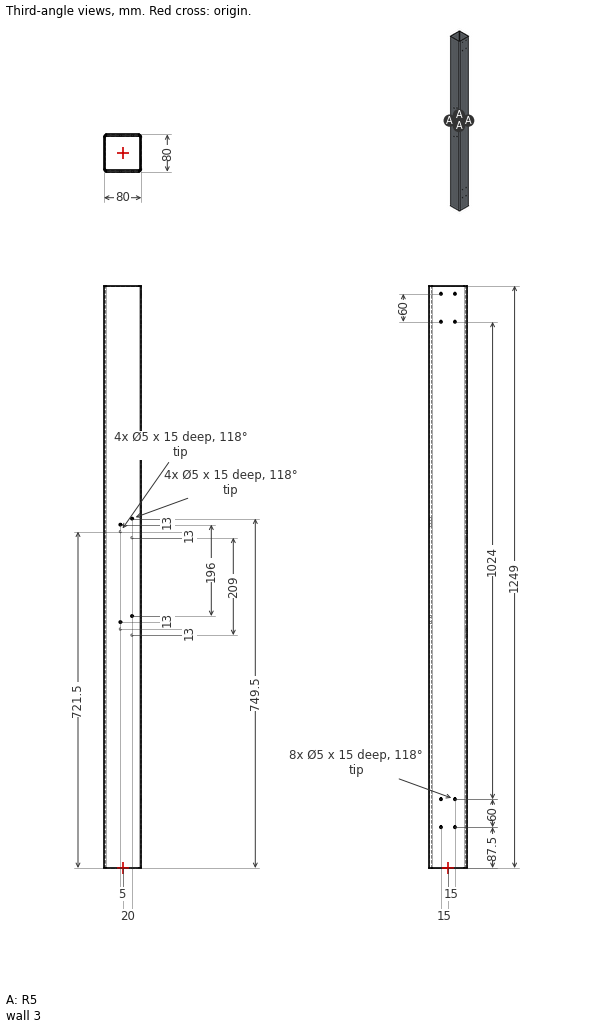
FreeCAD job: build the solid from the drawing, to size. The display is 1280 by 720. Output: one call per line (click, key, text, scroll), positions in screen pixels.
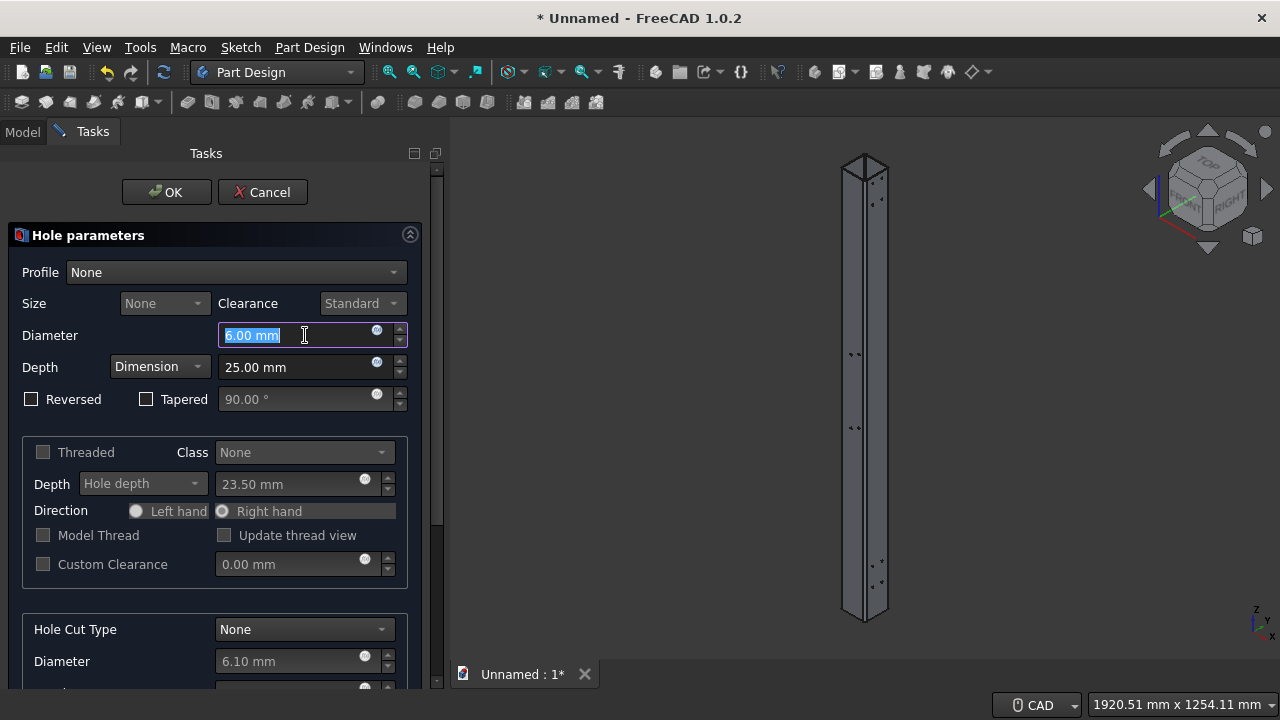
text(5)
key(Tab)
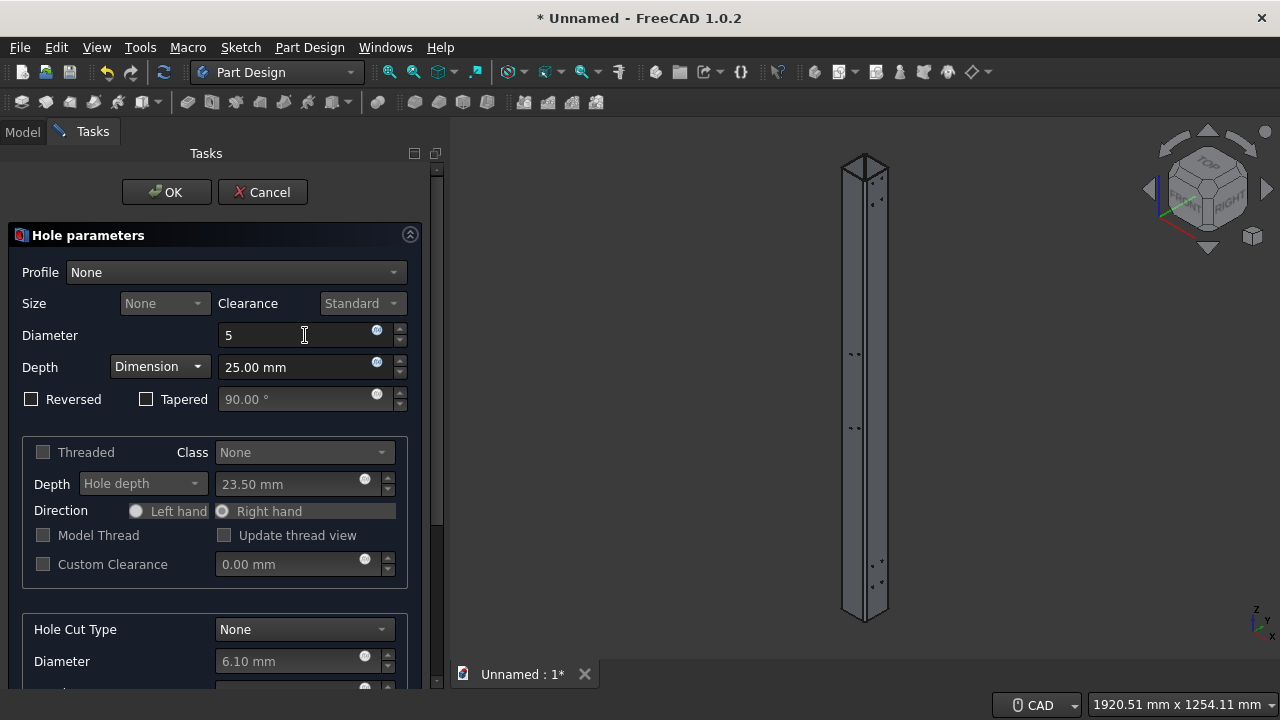
triple_click(305, 367)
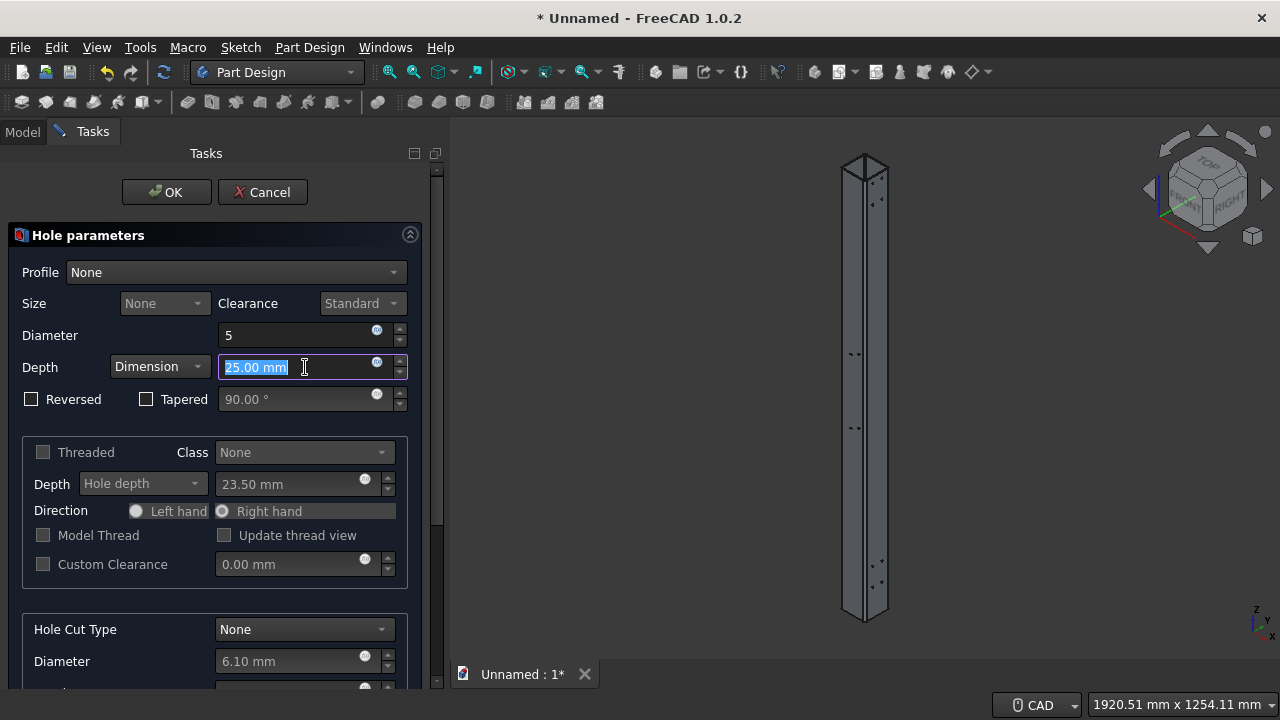
text(15)
key(Tab)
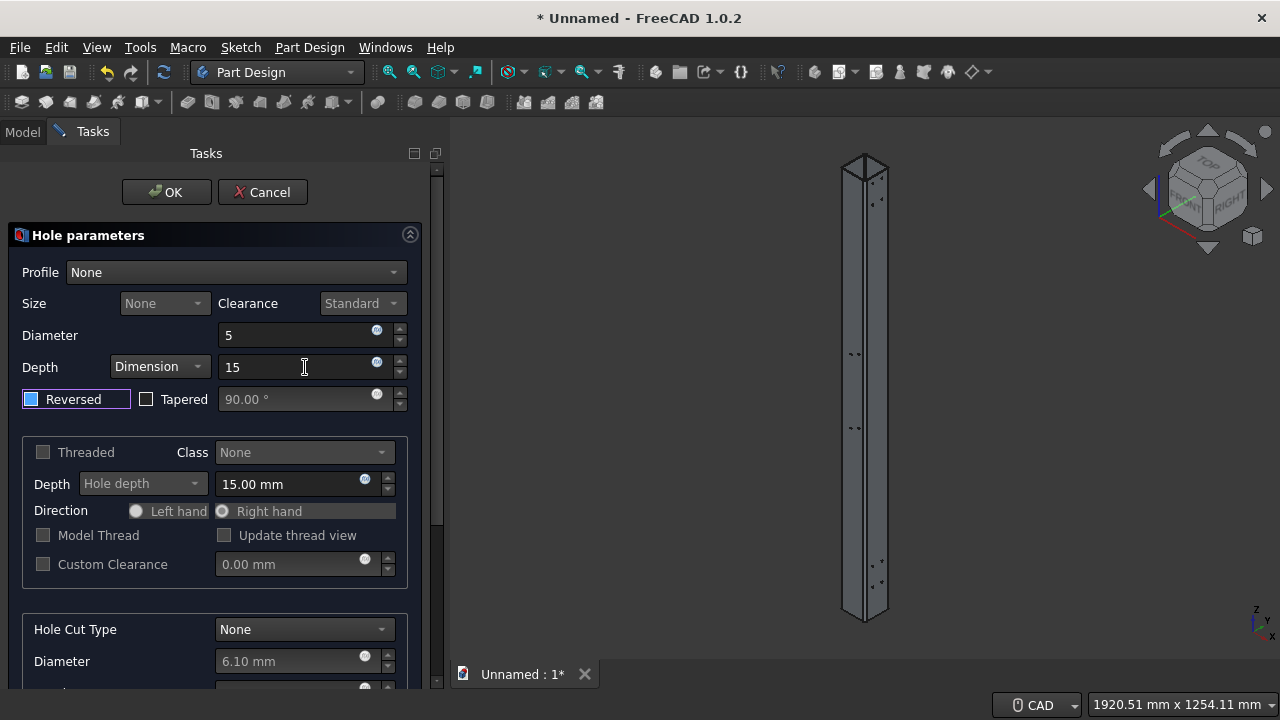
click(167, 192)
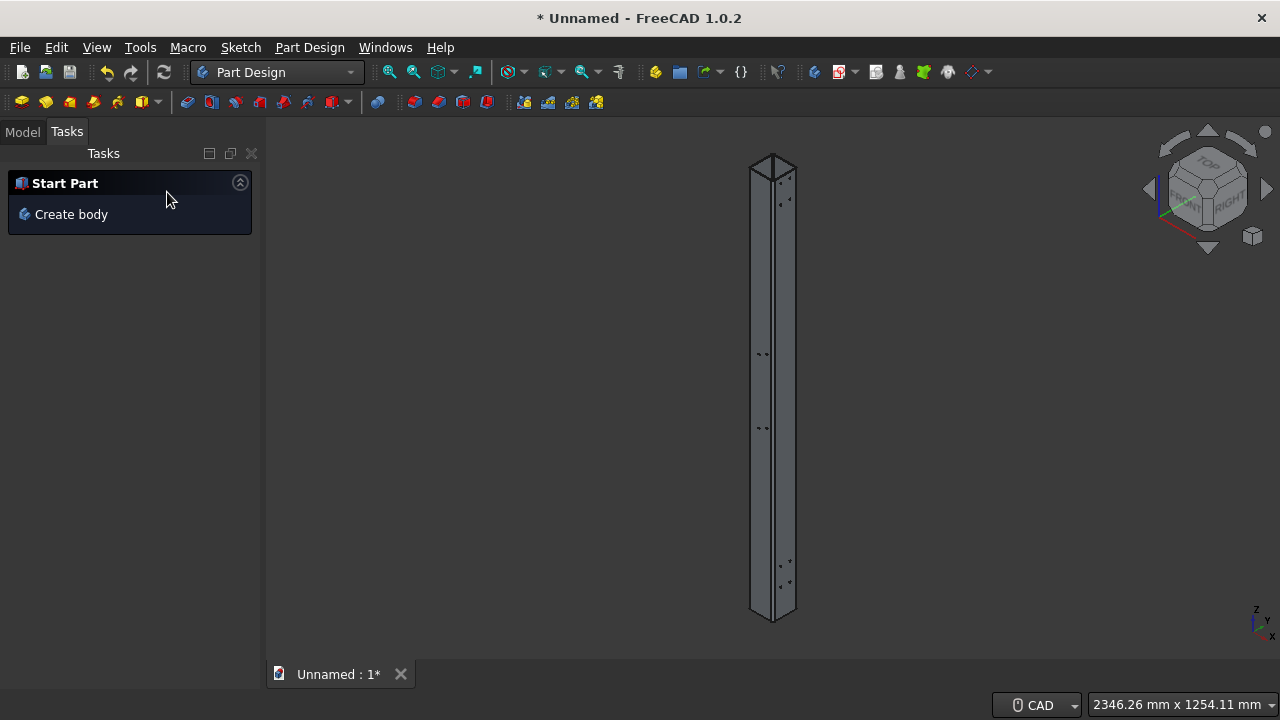
key(4)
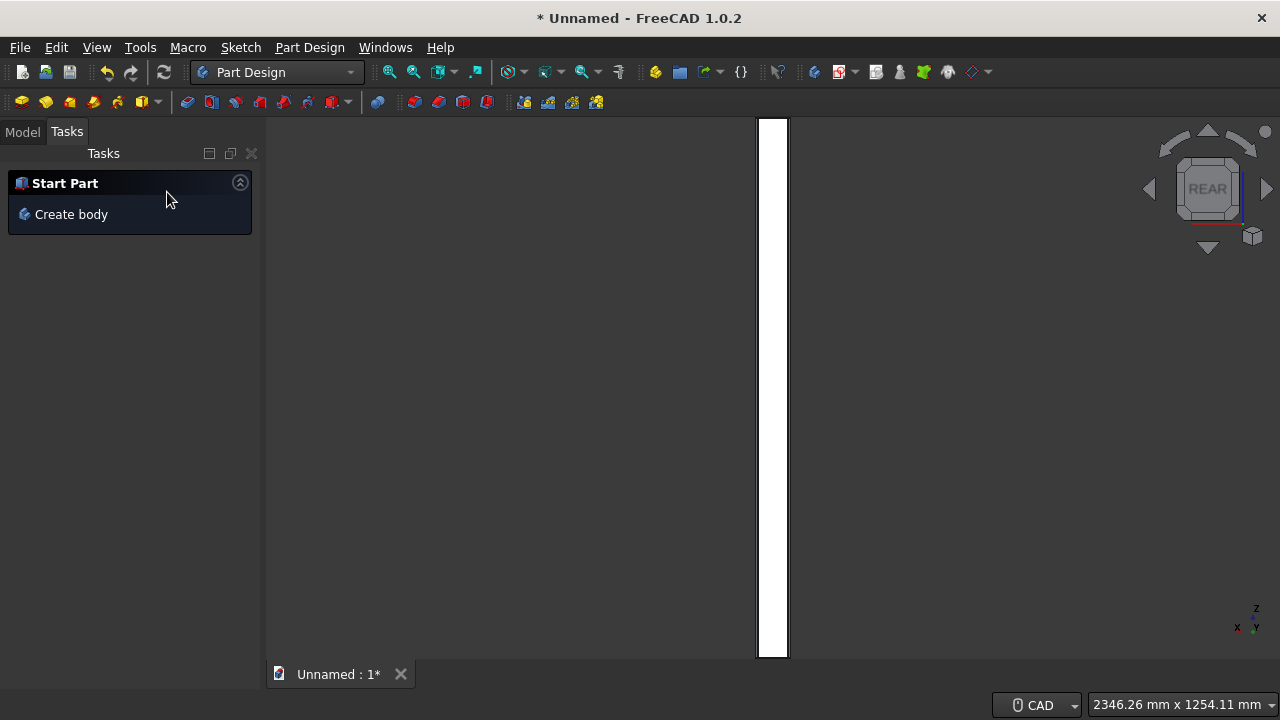
click(773, 156)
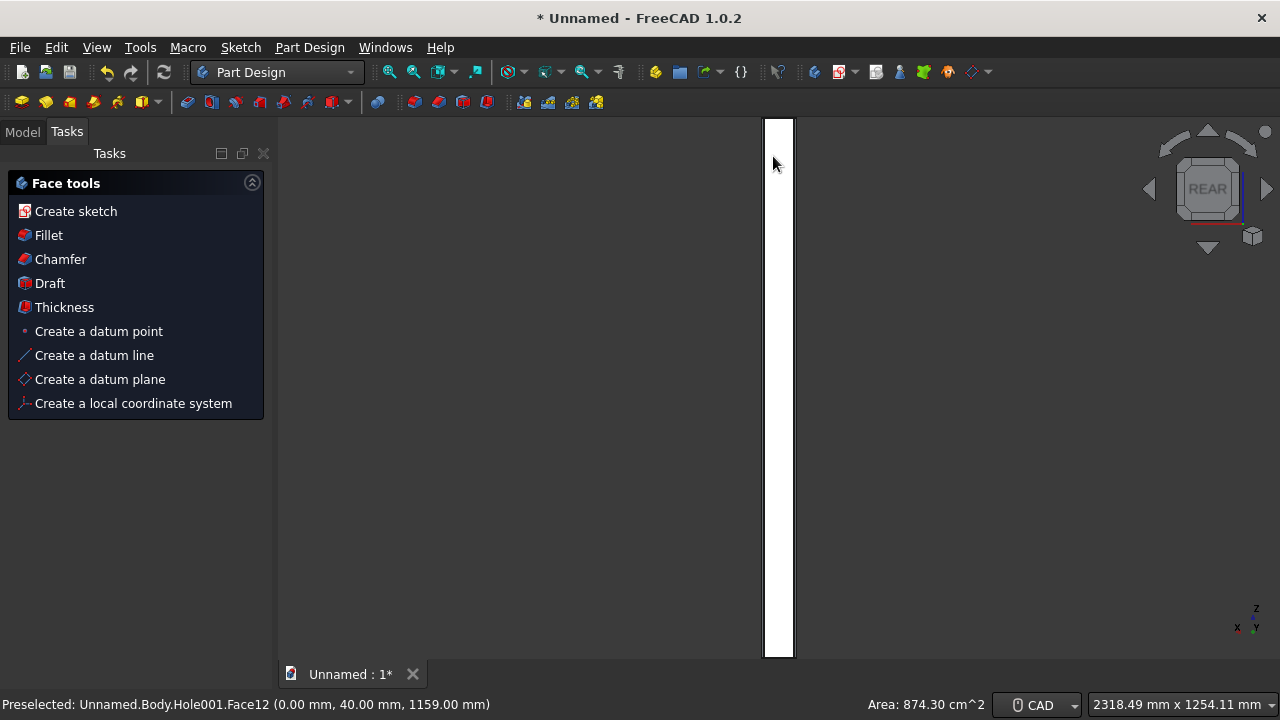
click(840, 72)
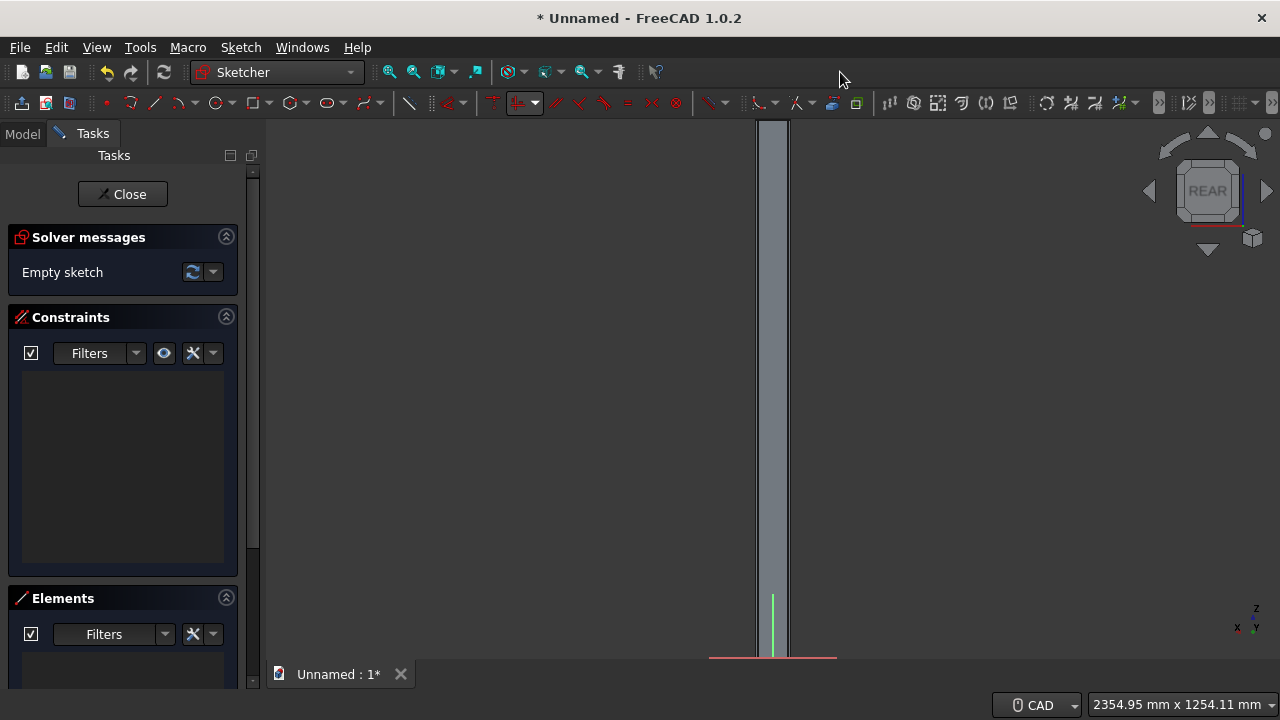
scroll(798, 398, up, 6)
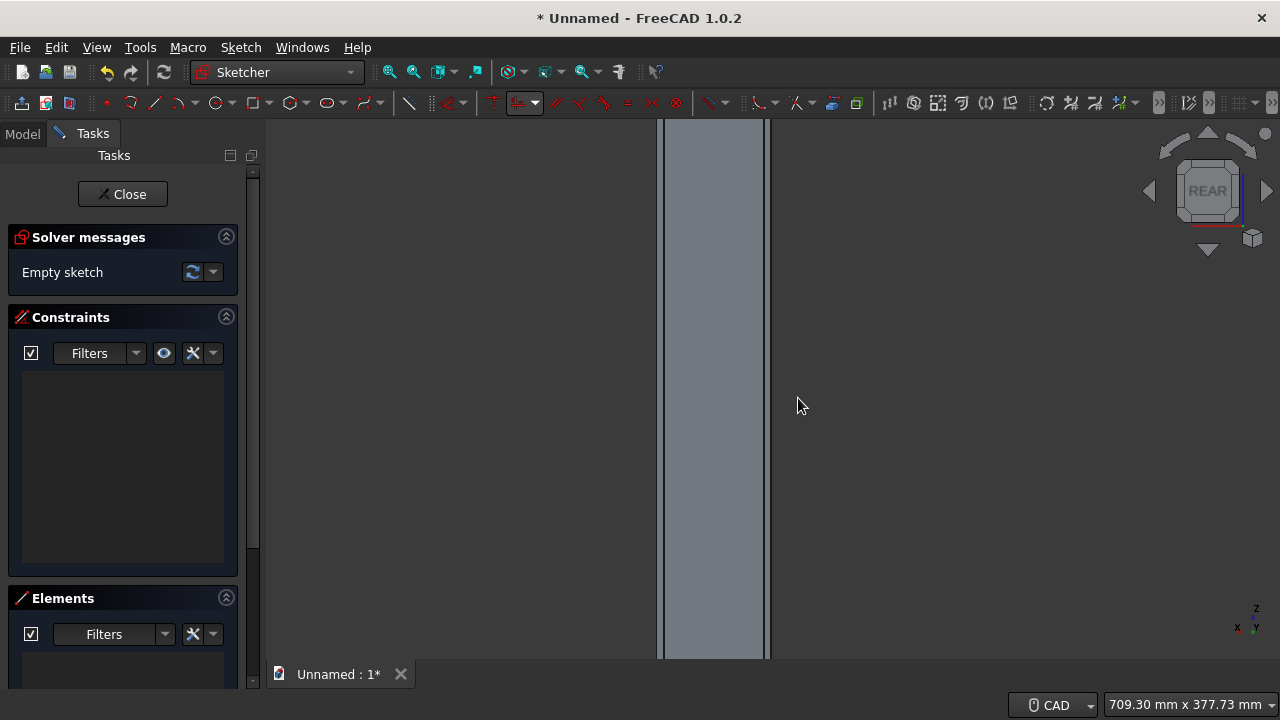
key(g)
key(c)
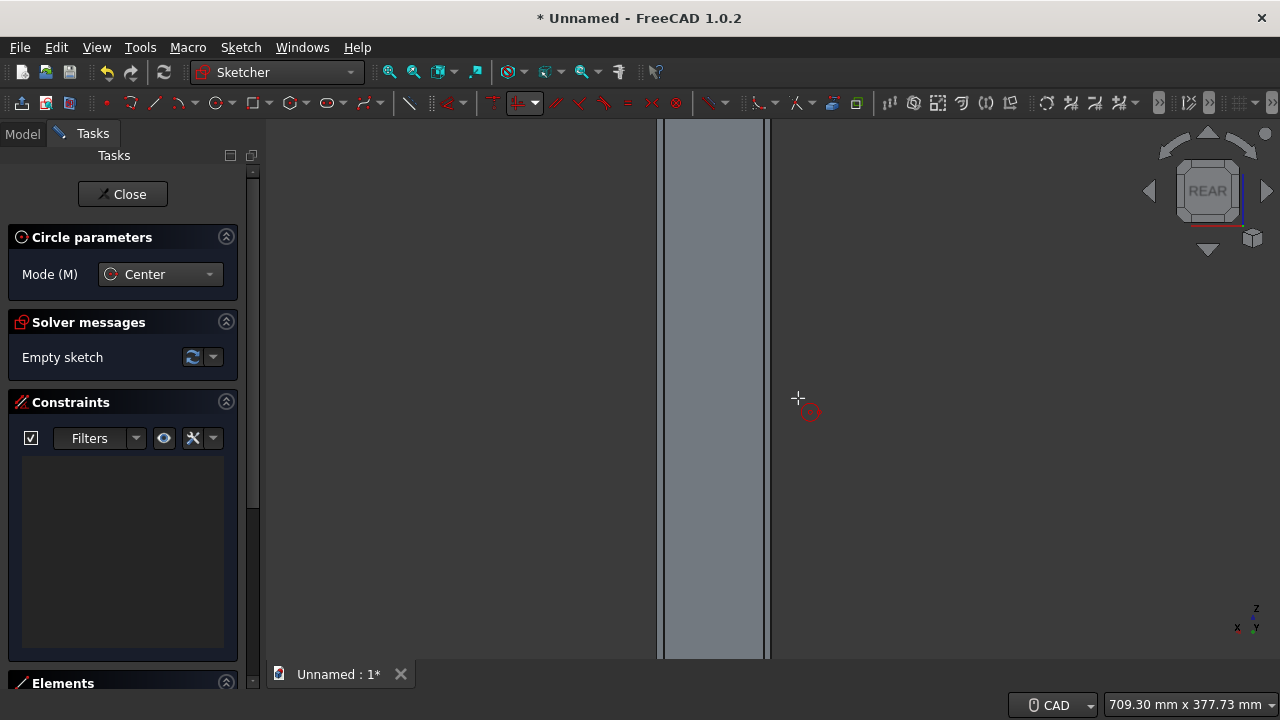
scroll(721, 228, up, 10)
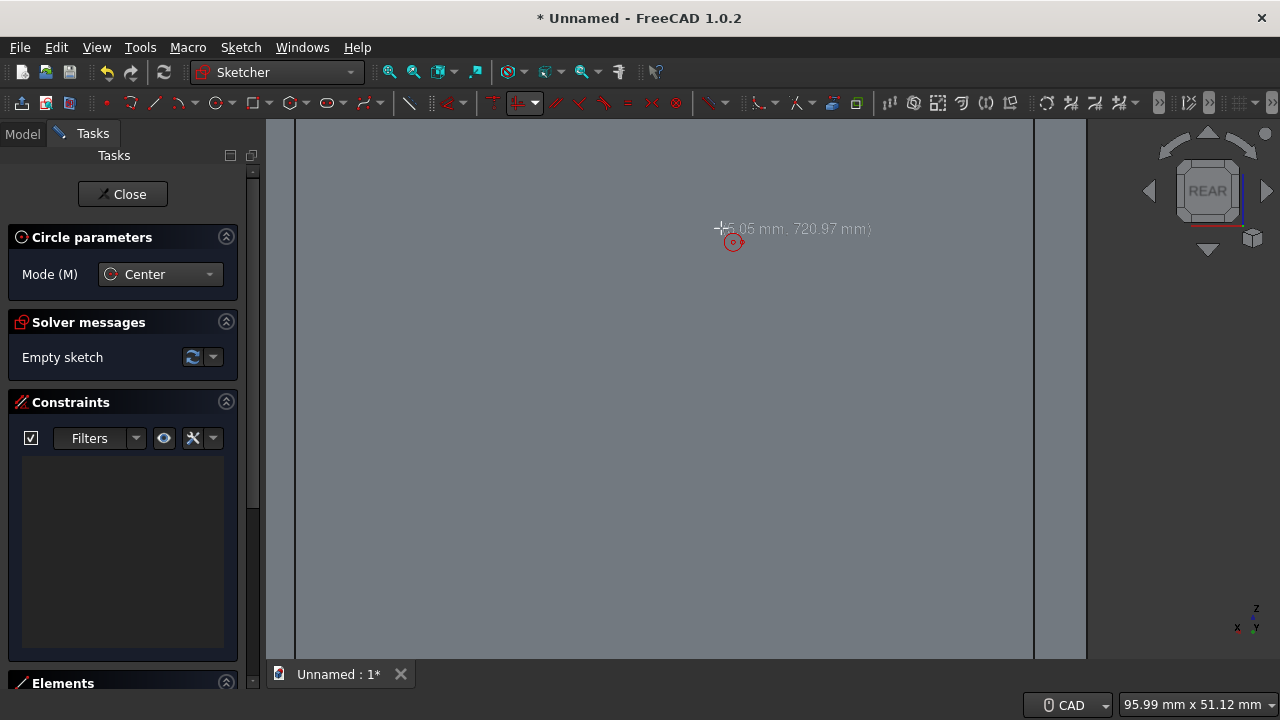
scroll(723, 231, down, 10)